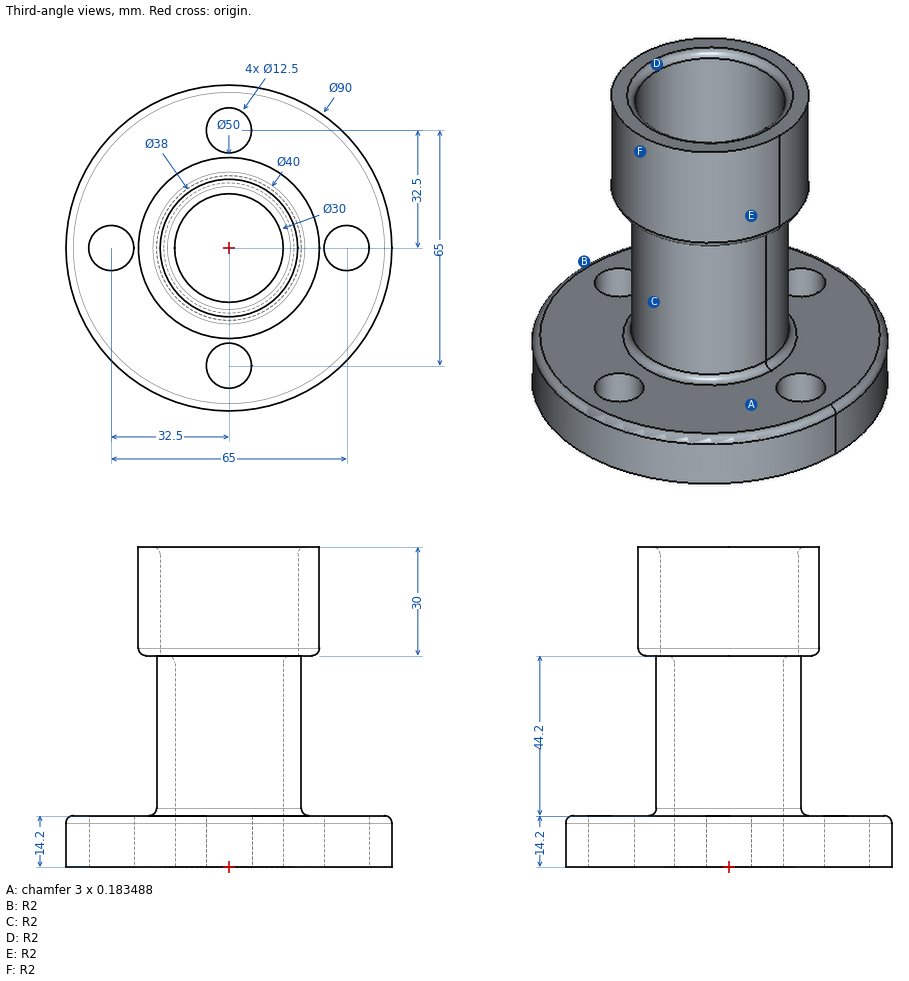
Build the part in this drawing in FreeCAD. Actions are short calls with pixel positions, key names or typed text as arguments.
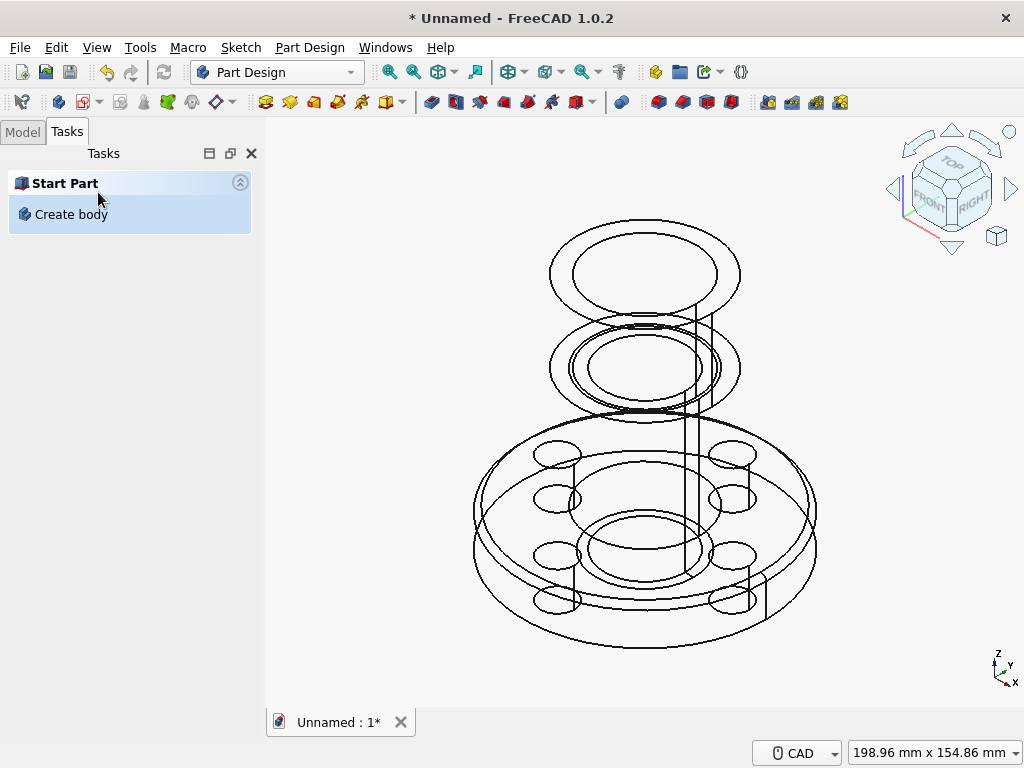
click(591, 473)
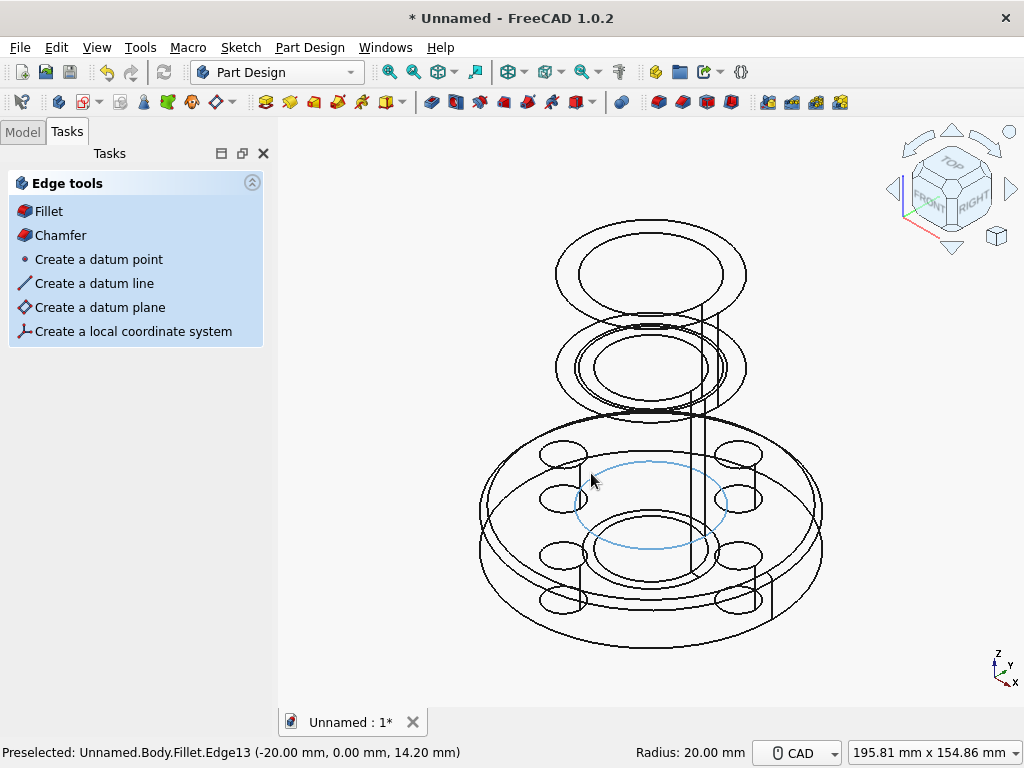
key(v)
key(1)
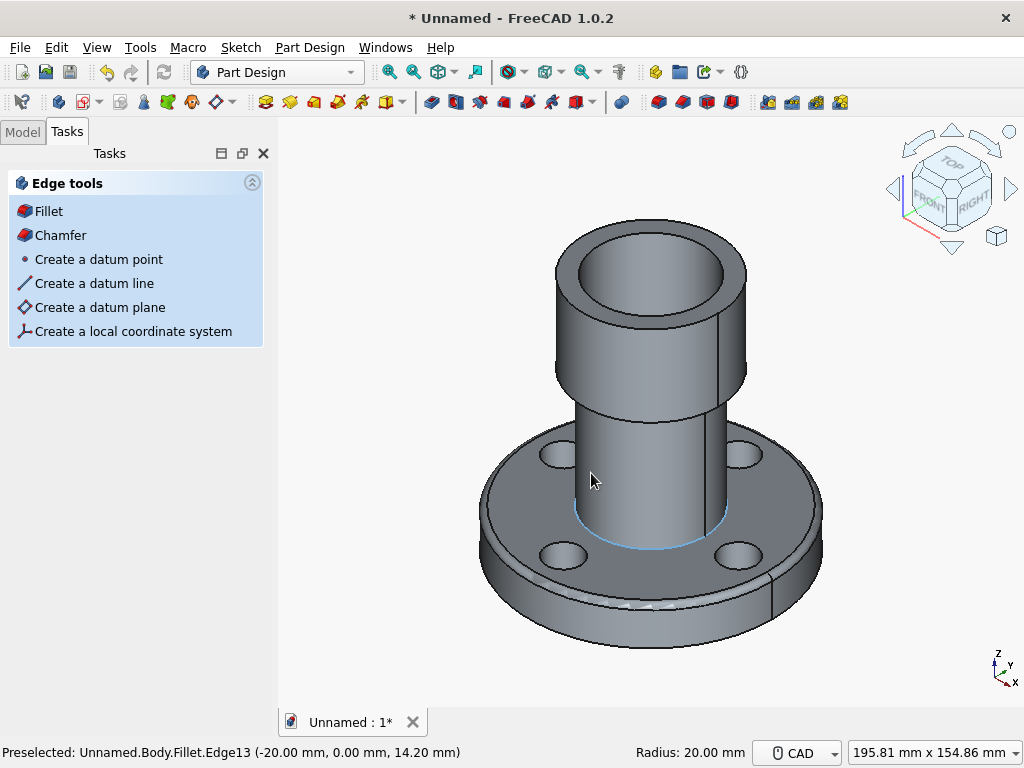
click(660, 102)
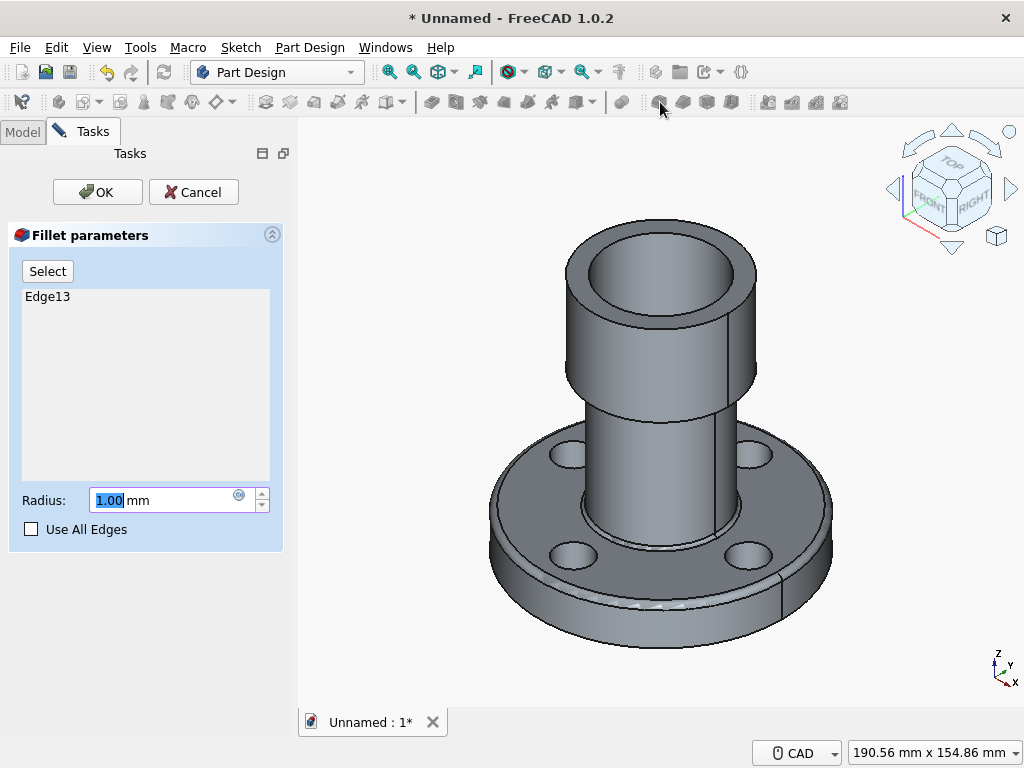
text(2)
key(Tab)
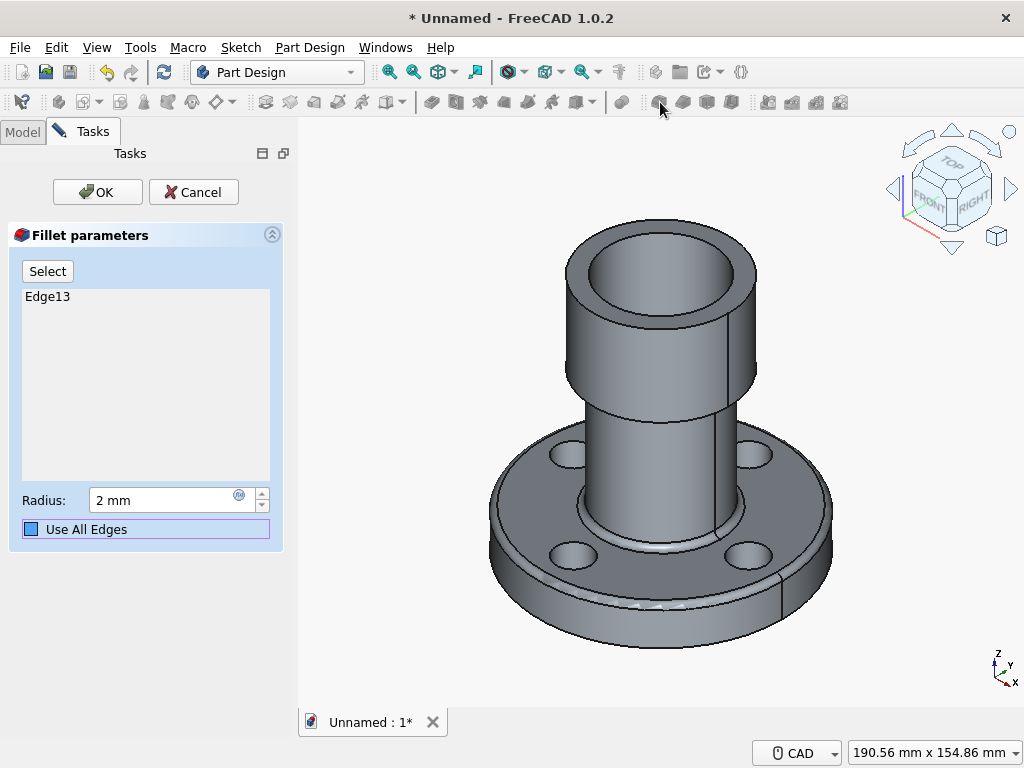
click(98, 192)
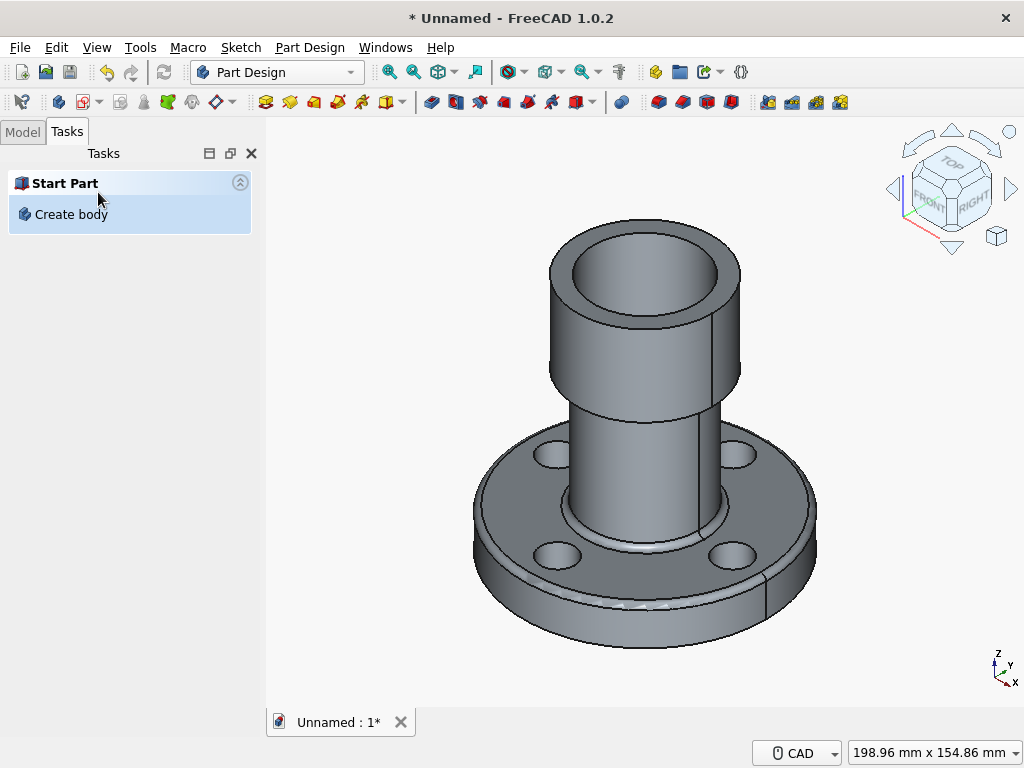
click(594, 244)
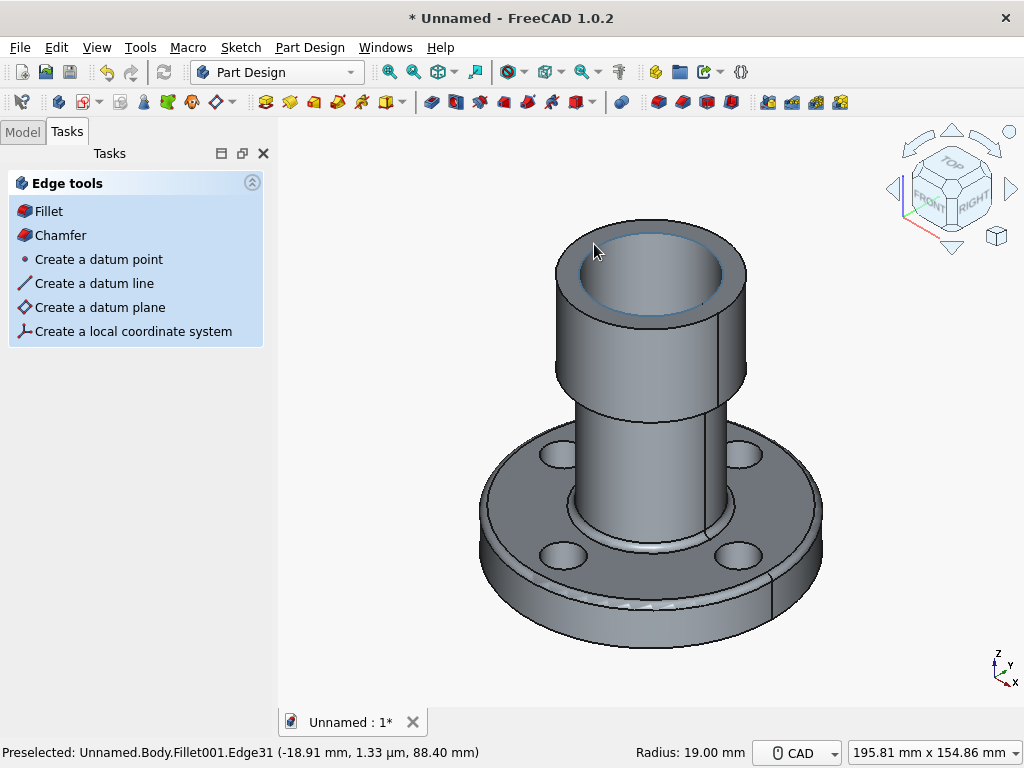
click(660, 102)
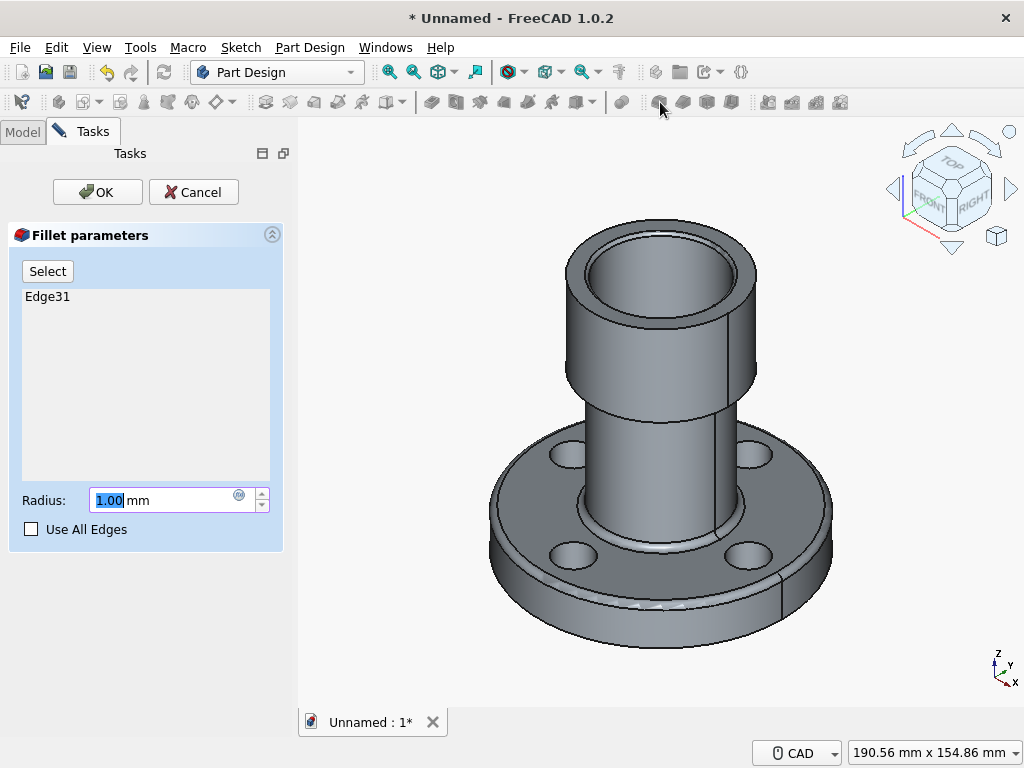
text(2)
key(Tab)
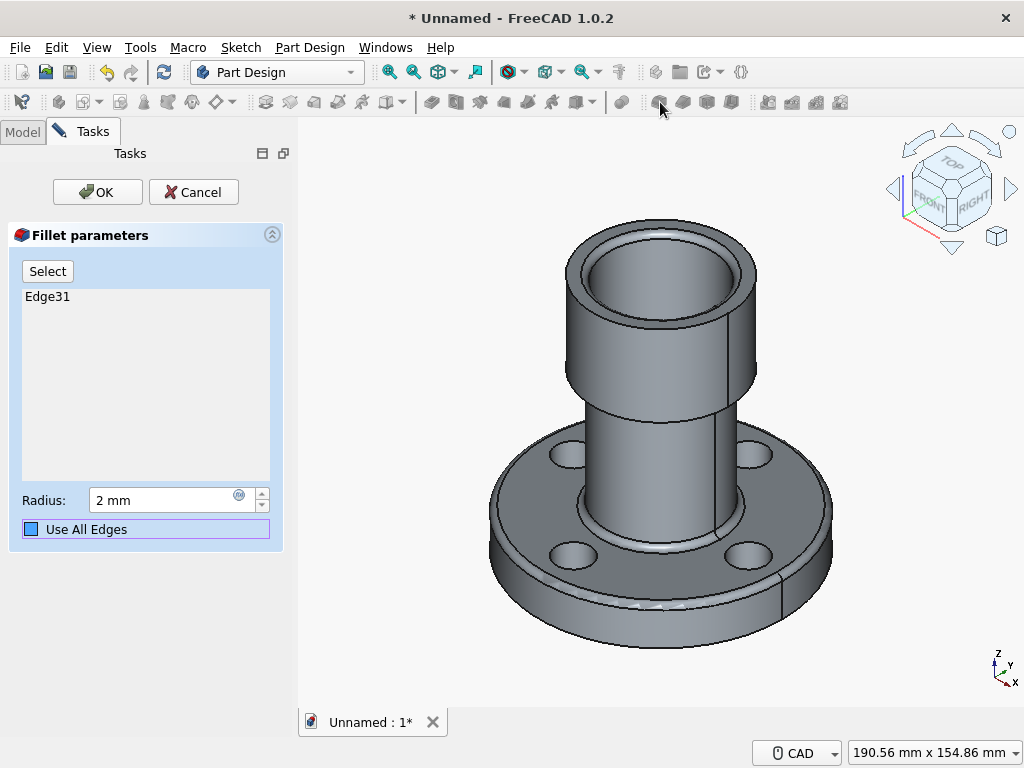
click(98, 192)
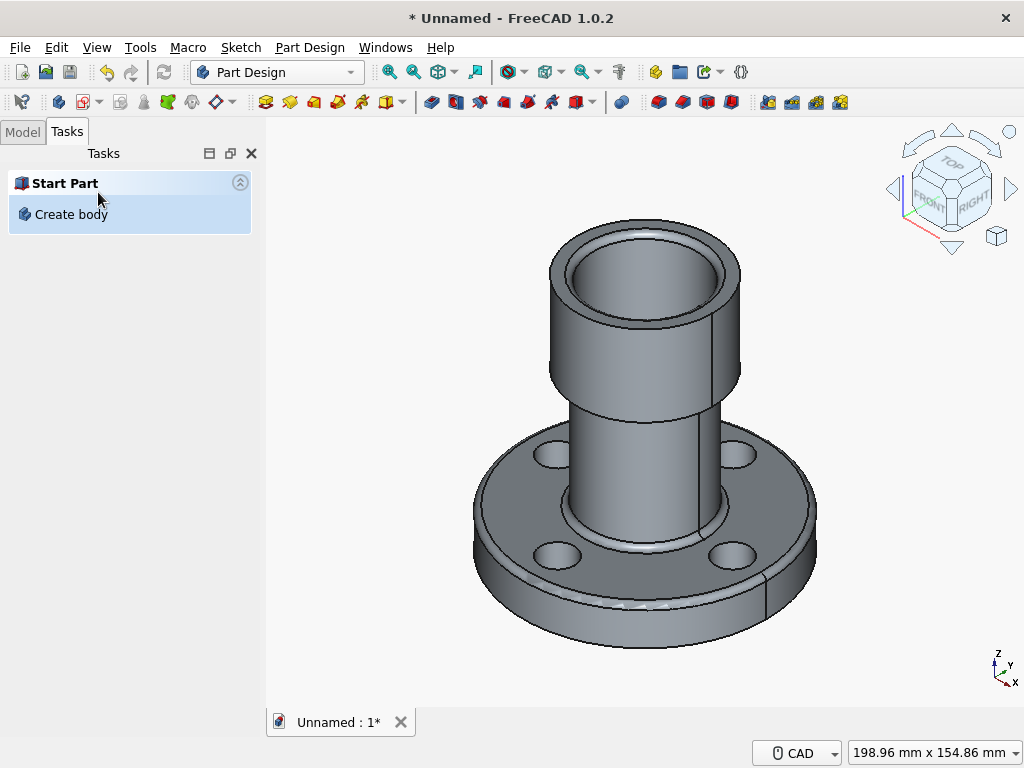
key(2)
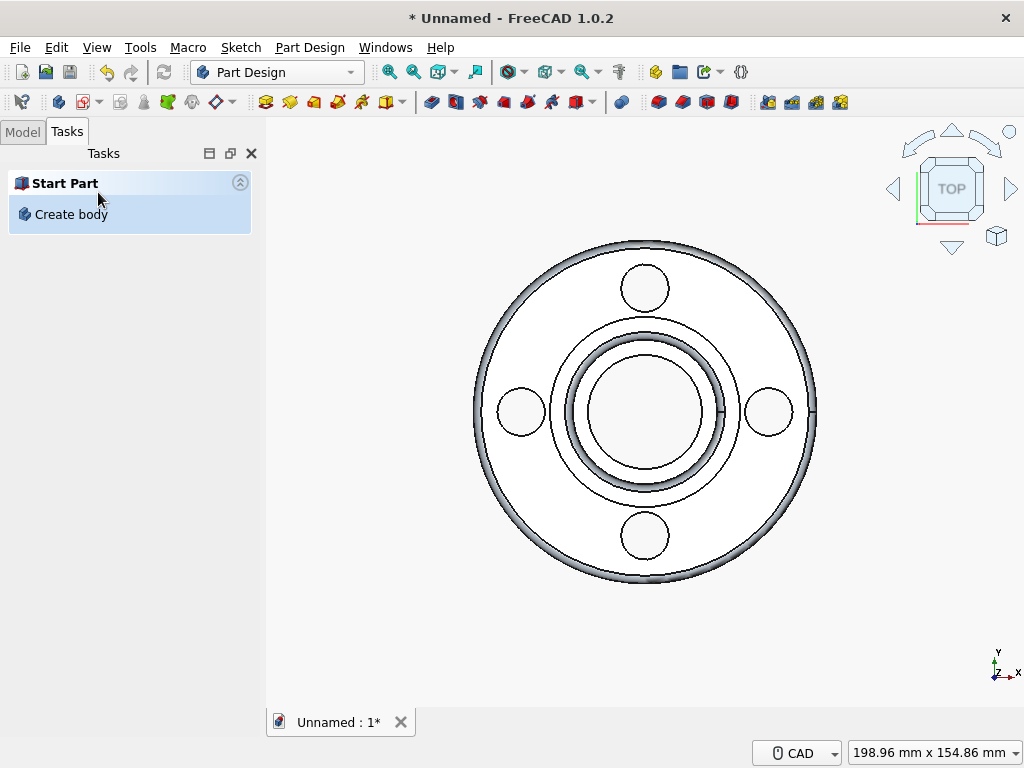
click(588, 411)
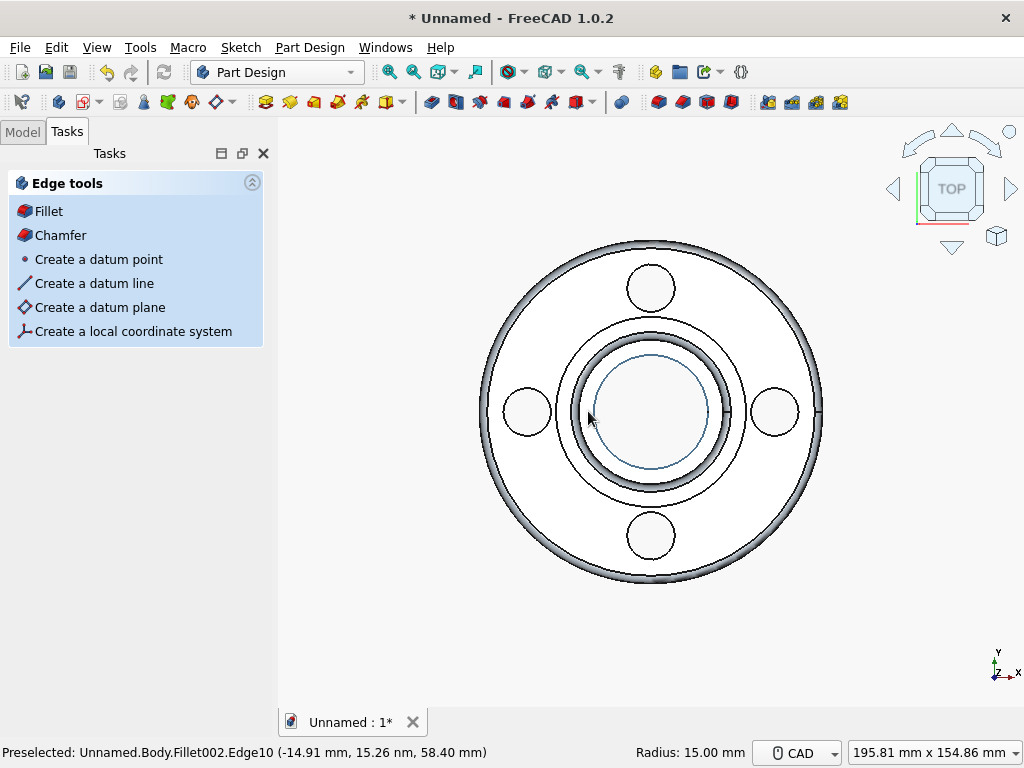
click(660, 102)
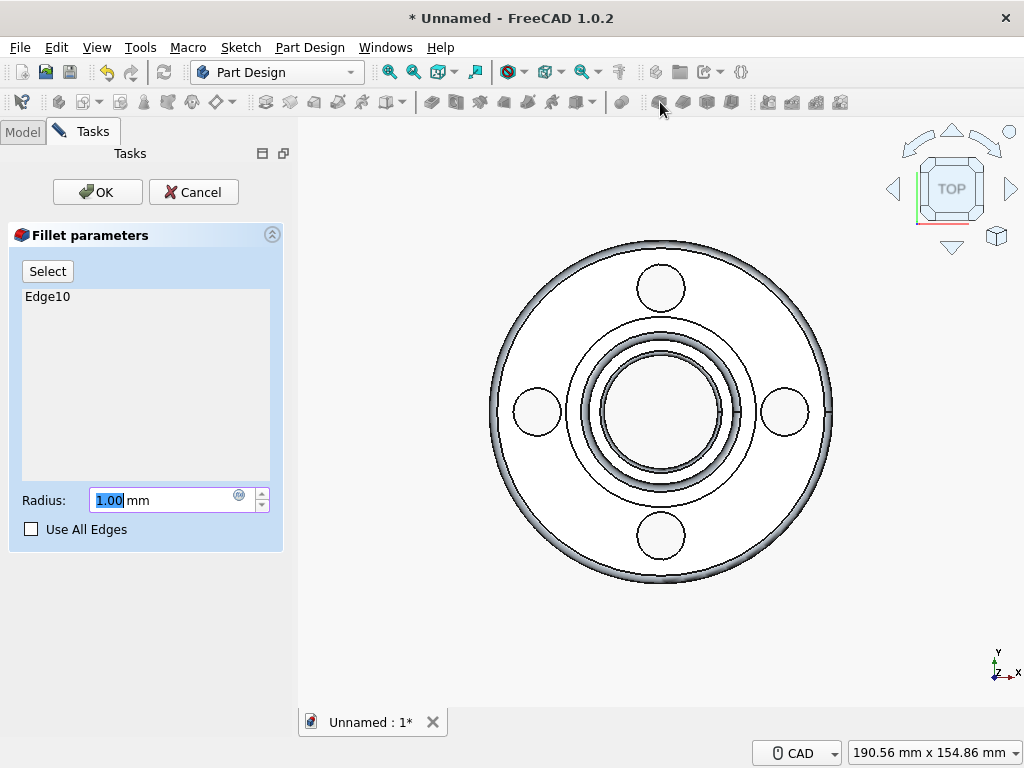
text(2)
key(Tab)